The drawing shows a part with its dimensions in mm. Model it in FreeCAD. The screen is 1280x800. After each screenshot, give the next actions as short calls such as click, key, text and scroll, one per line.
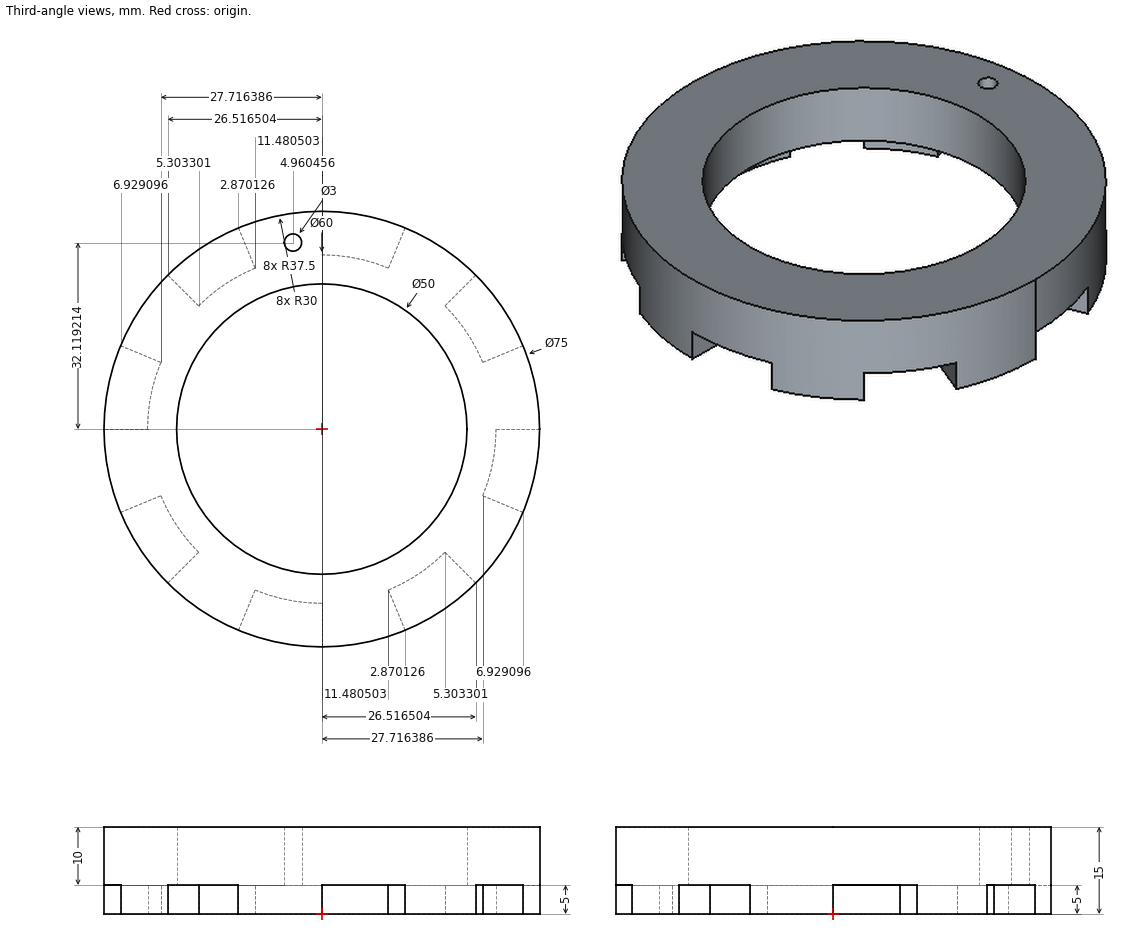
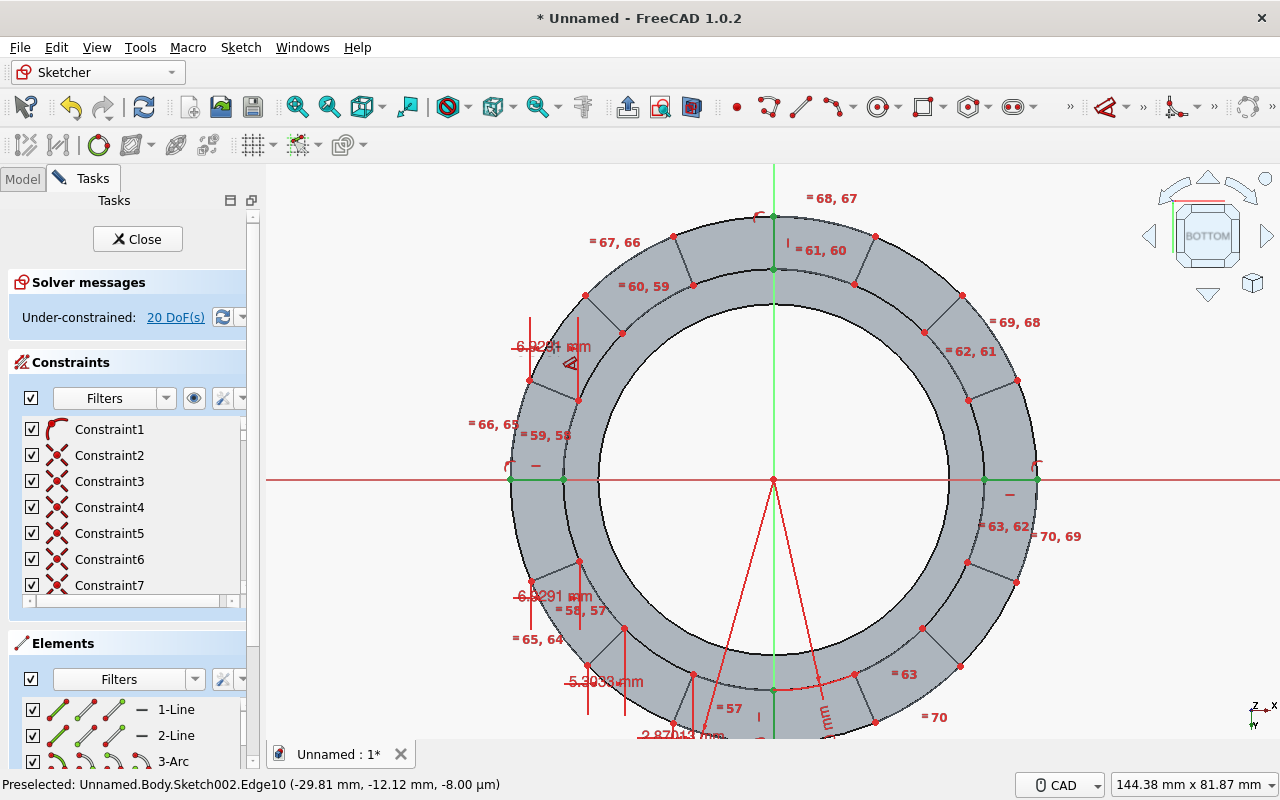
click(597, 307)
click(604, 262)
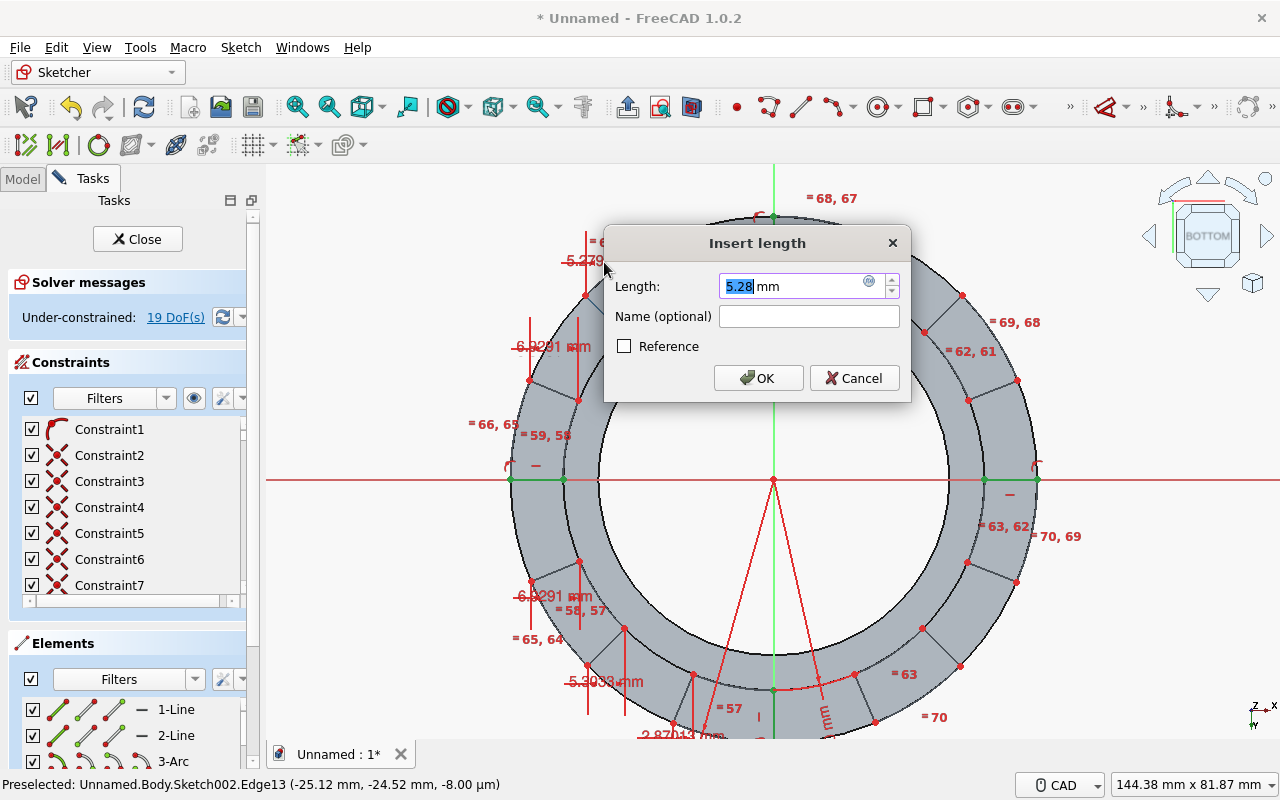
text(5.303301)
key(Return)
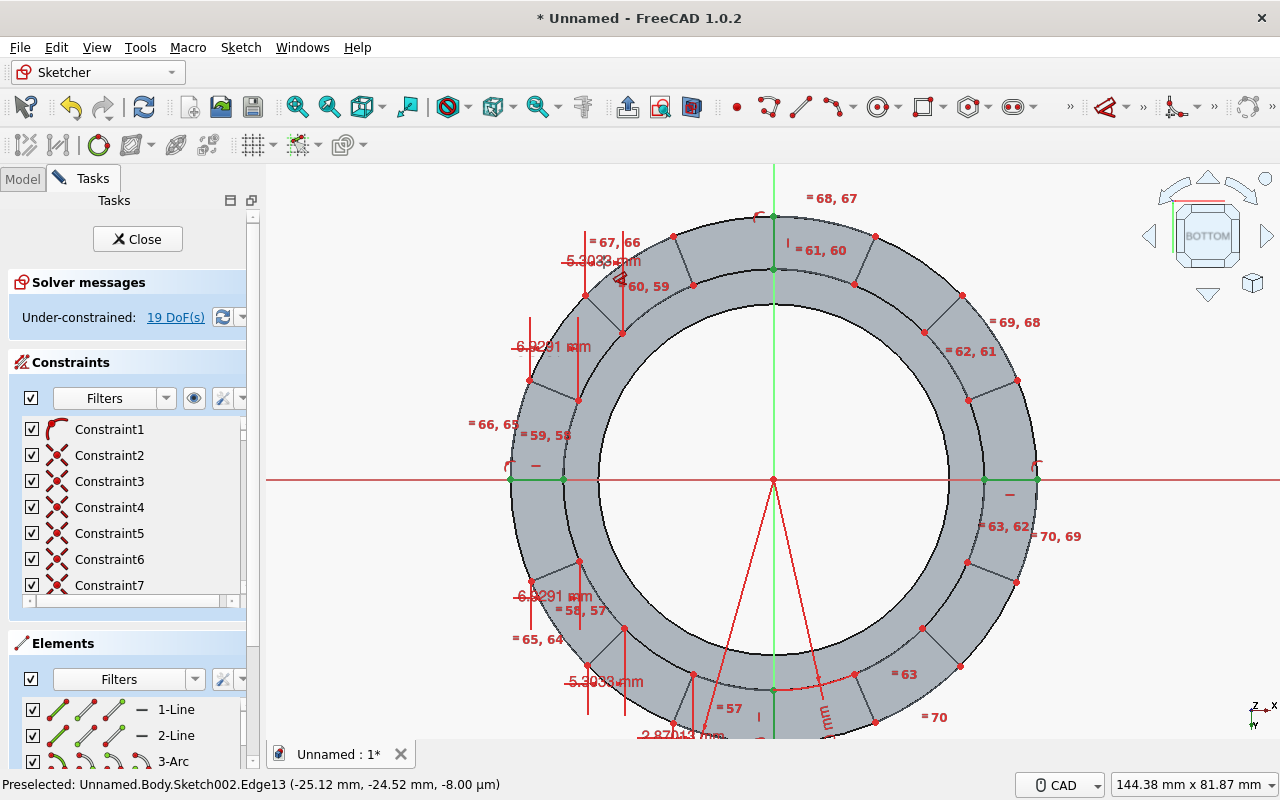
scroll(687, 270, up, 4)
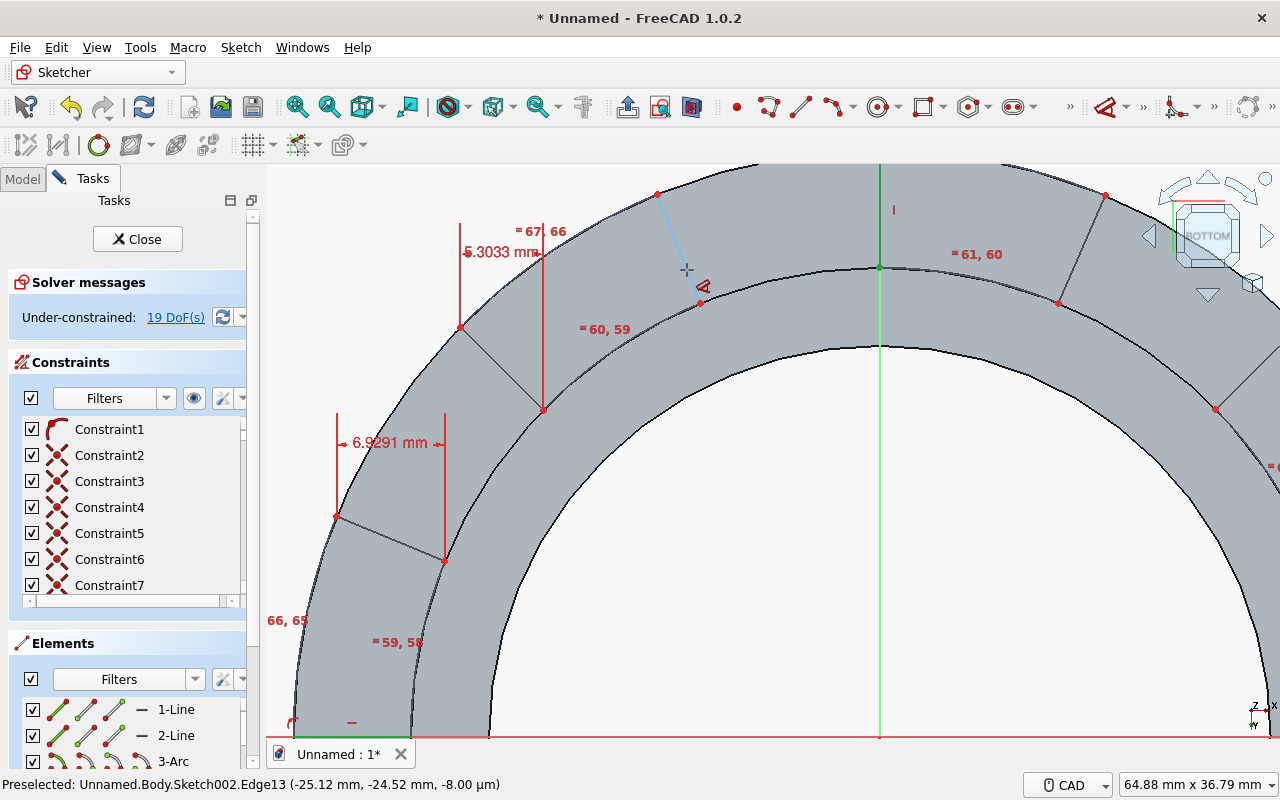
click(688, 271)
click(679, 337)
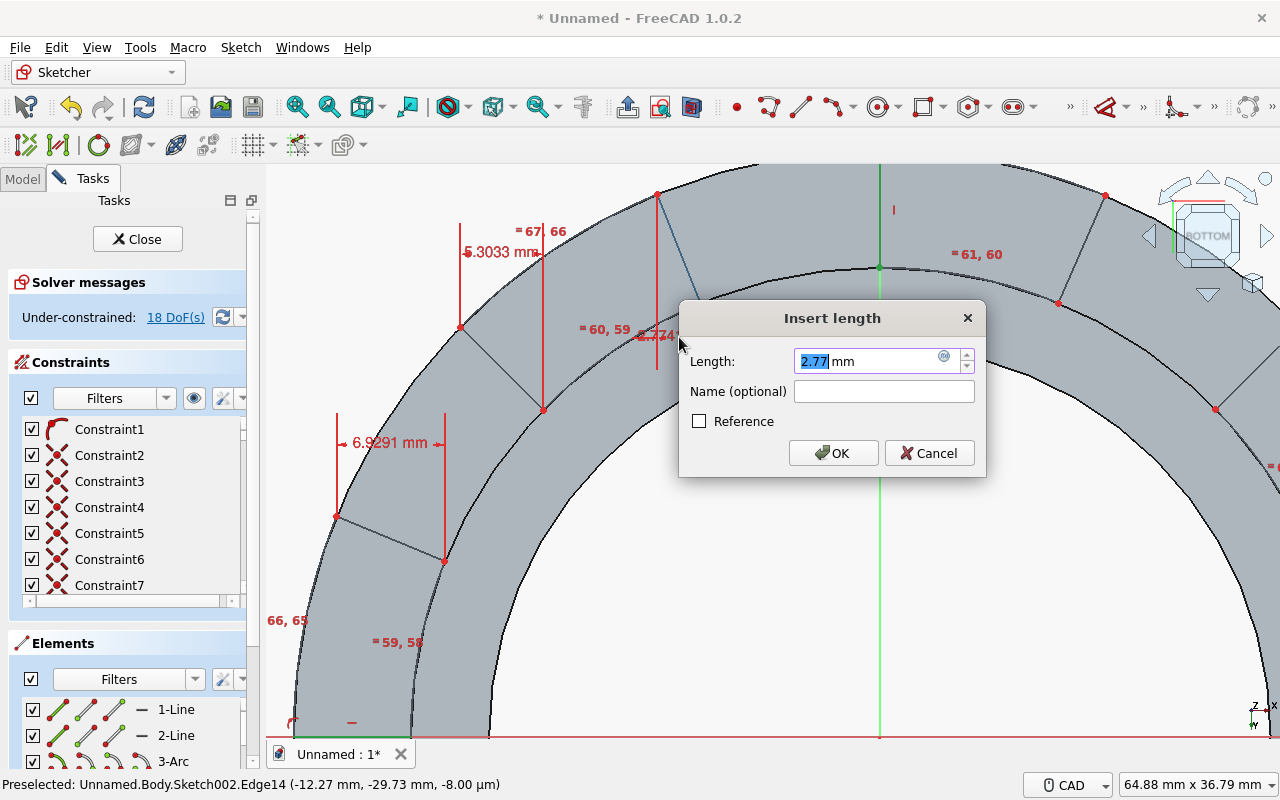
text(2.870126)
key(Return)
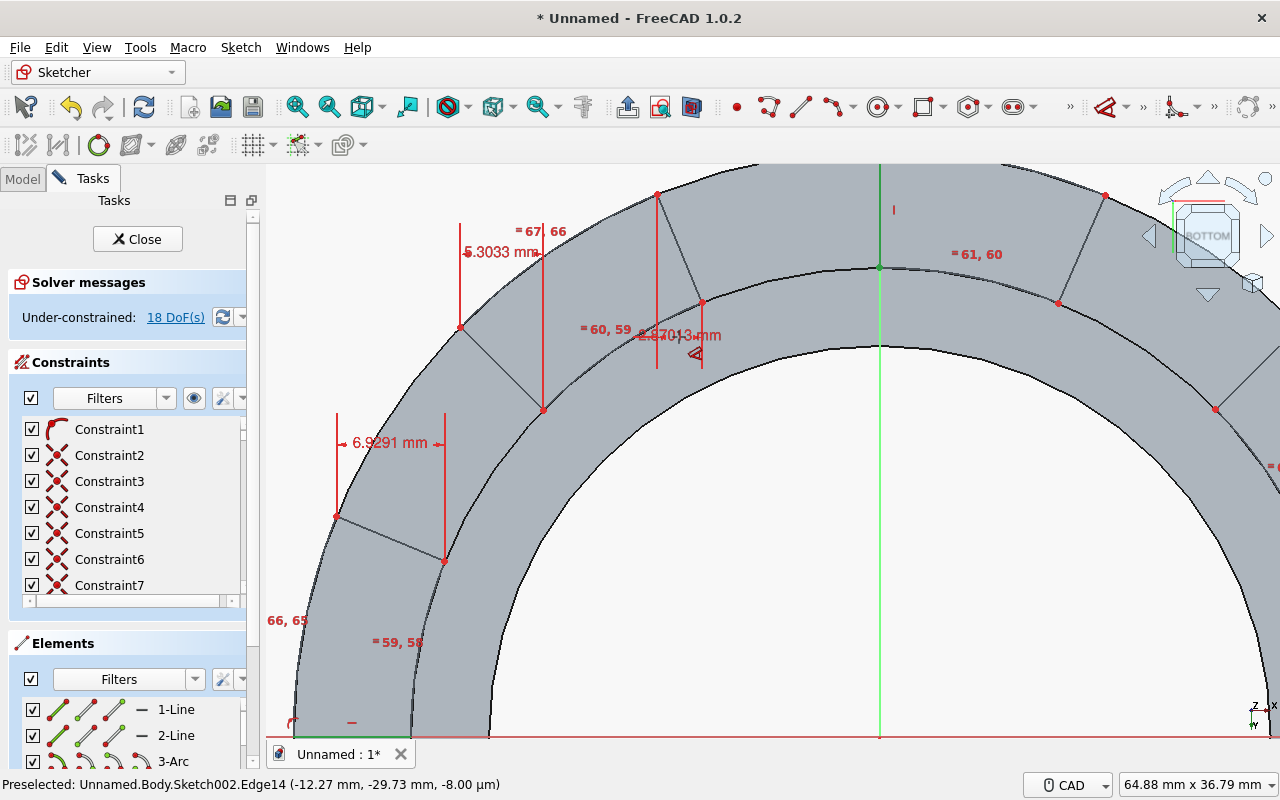
click(1072, 271)
click(1082, 337)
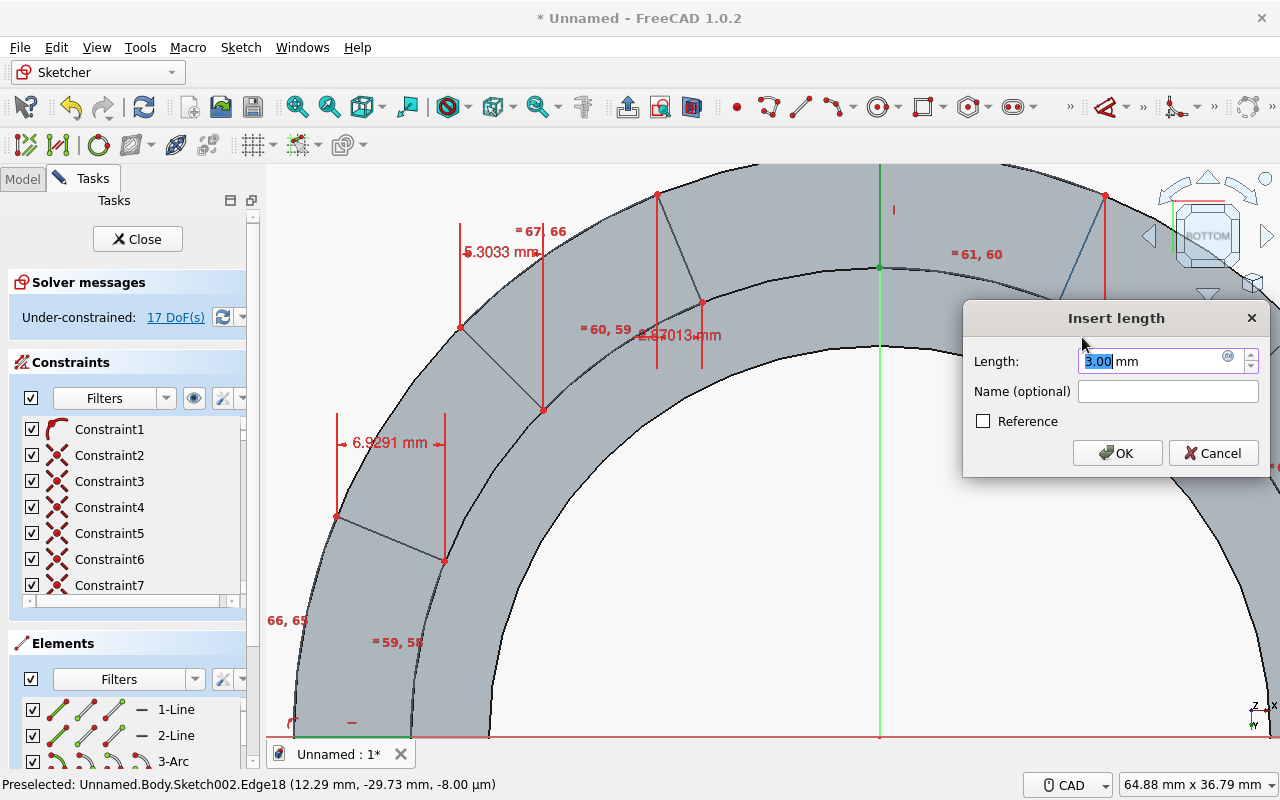
text(2.870126)
key(Return)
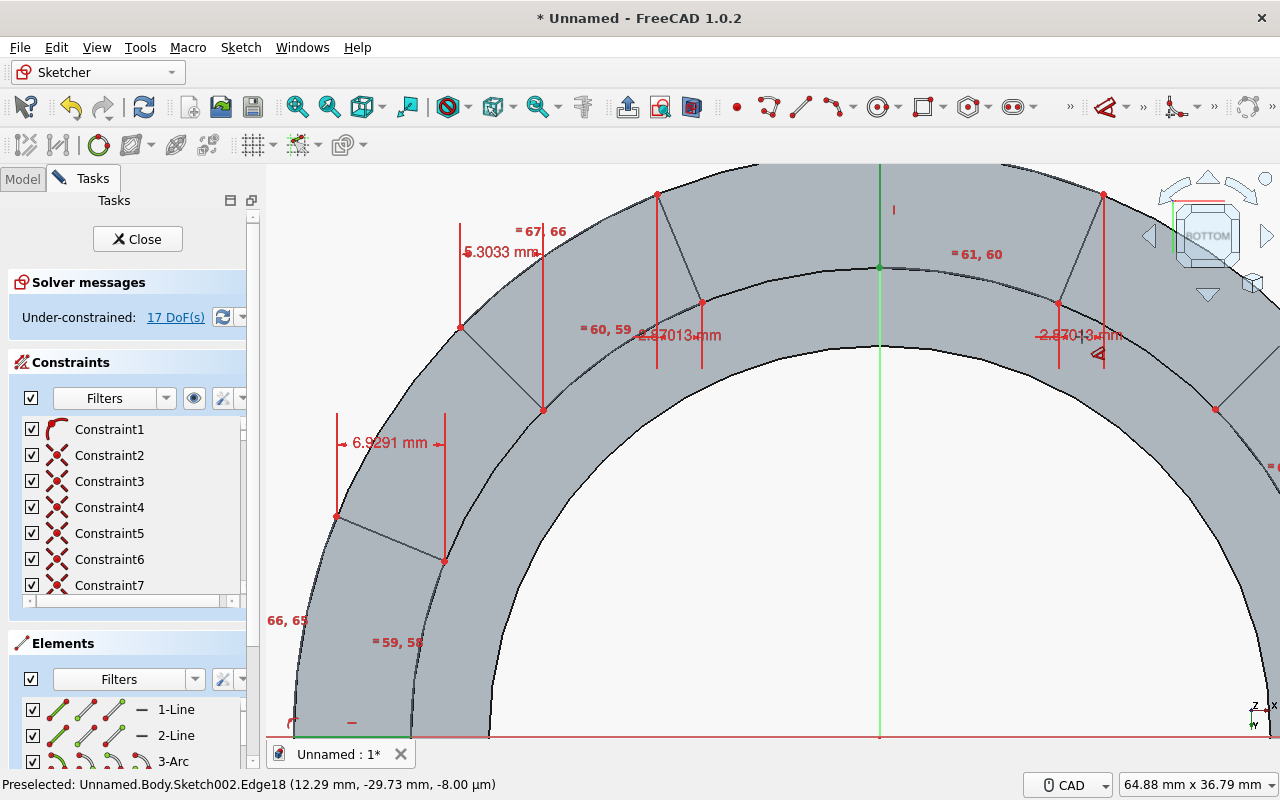
scroll(629, 329, down, 6)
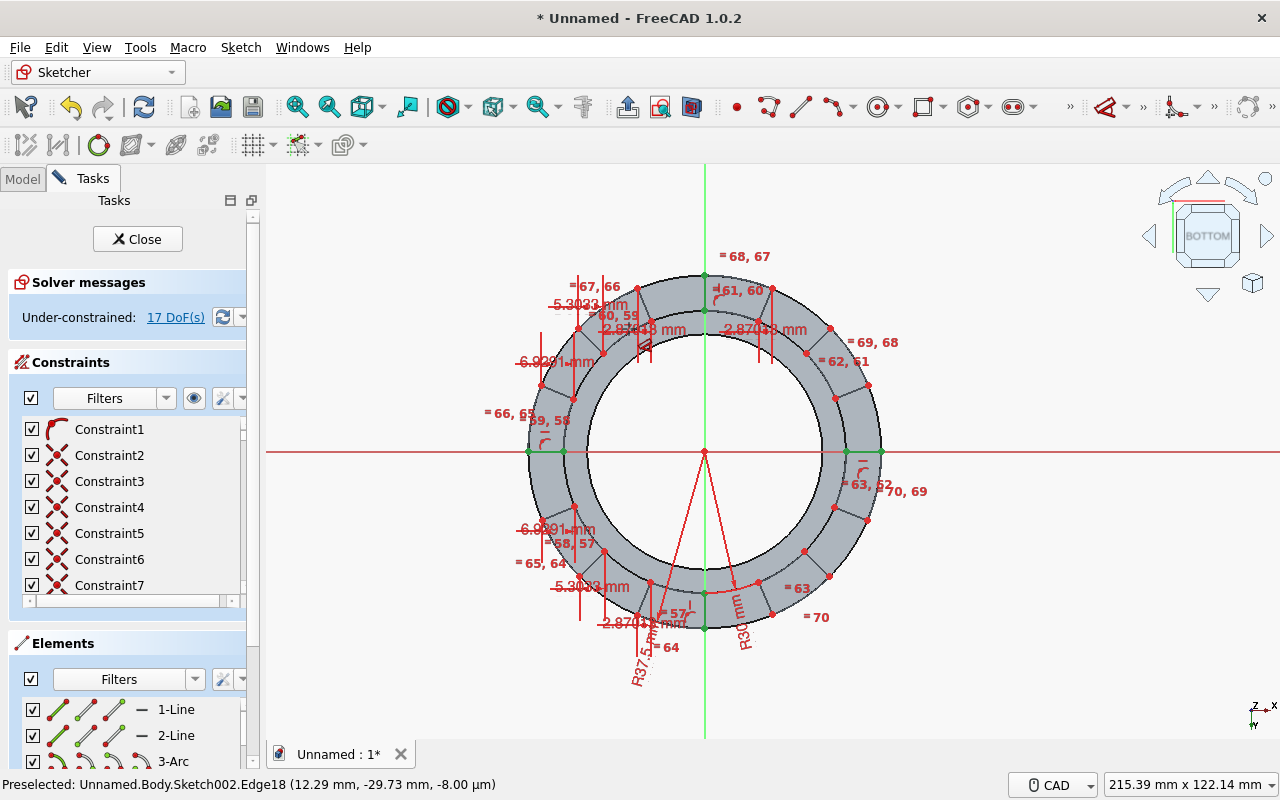
scroll(823, 336, up, 3)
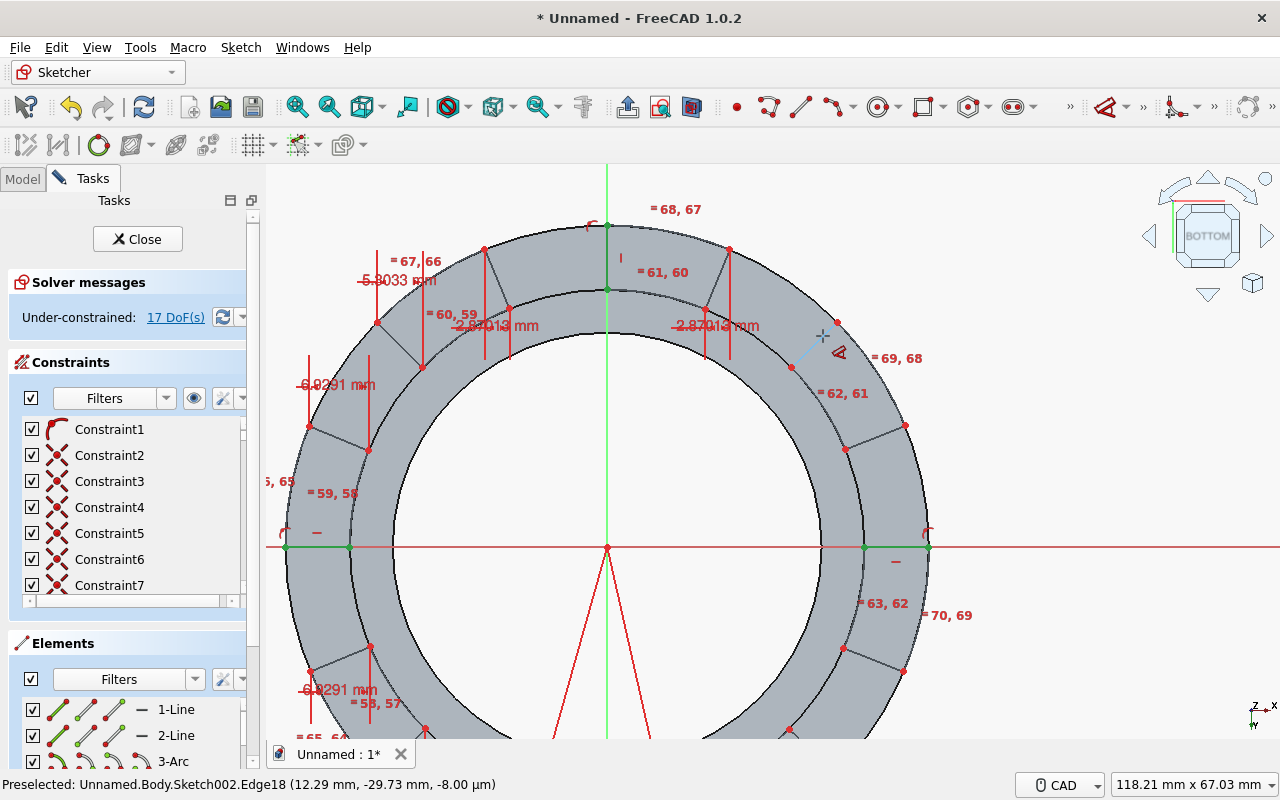
click(823, 336)
click(814, 288)